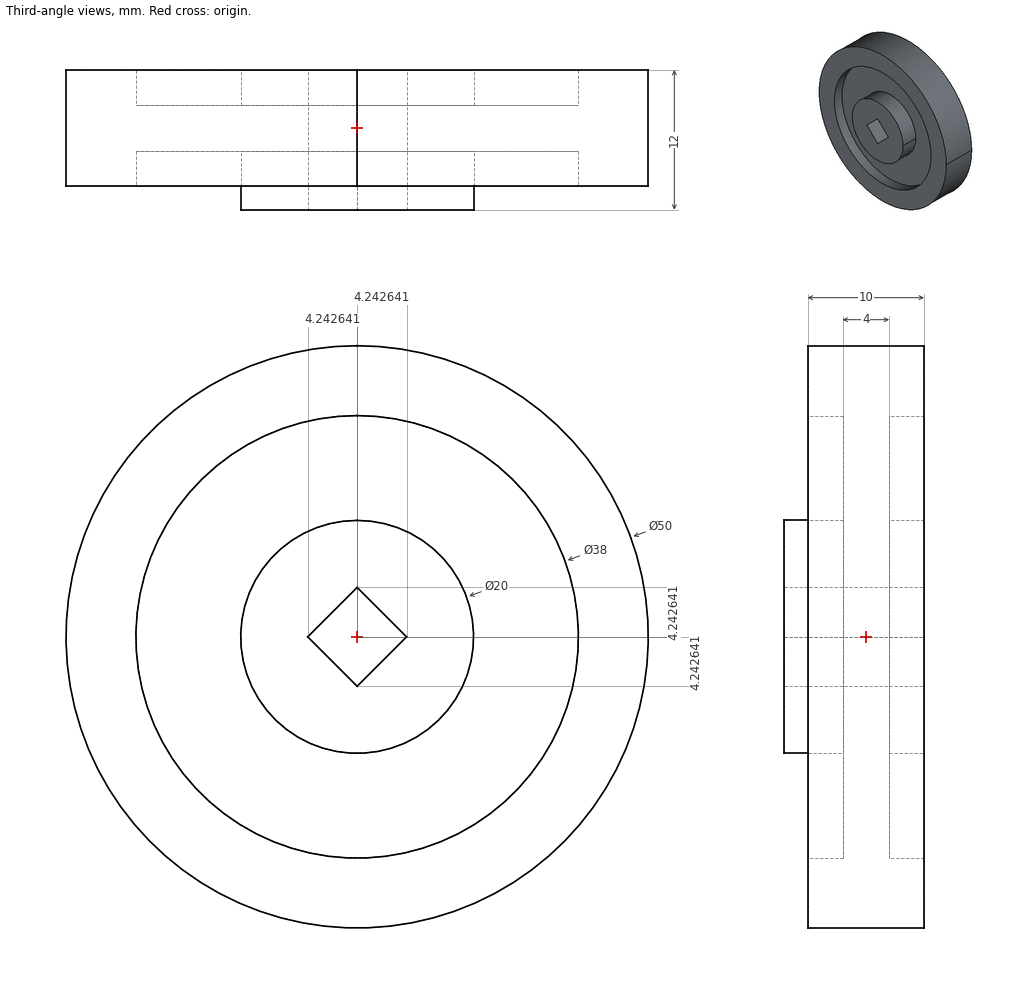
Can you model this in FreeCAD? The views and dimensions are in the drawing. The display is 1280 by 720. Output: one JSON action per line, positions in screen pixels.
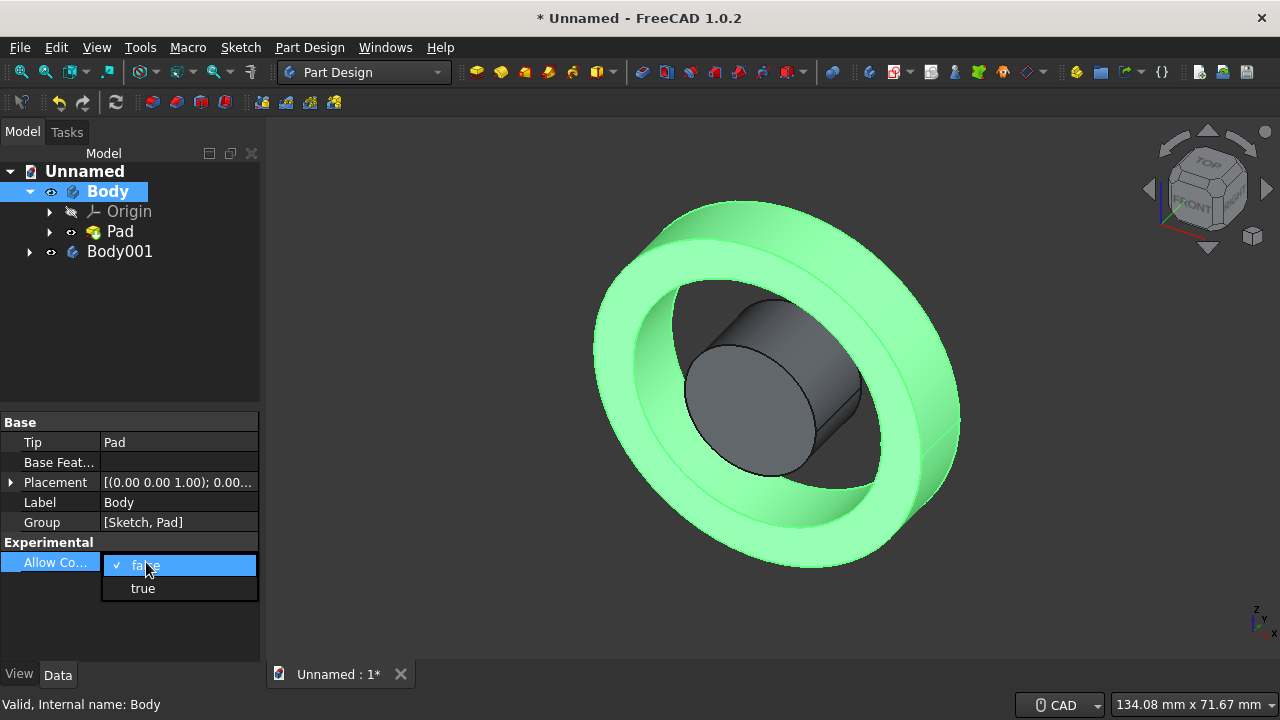
{"action": "left_click", "coordinate": [179, 588]}
{"action": "key", "text": "Return"}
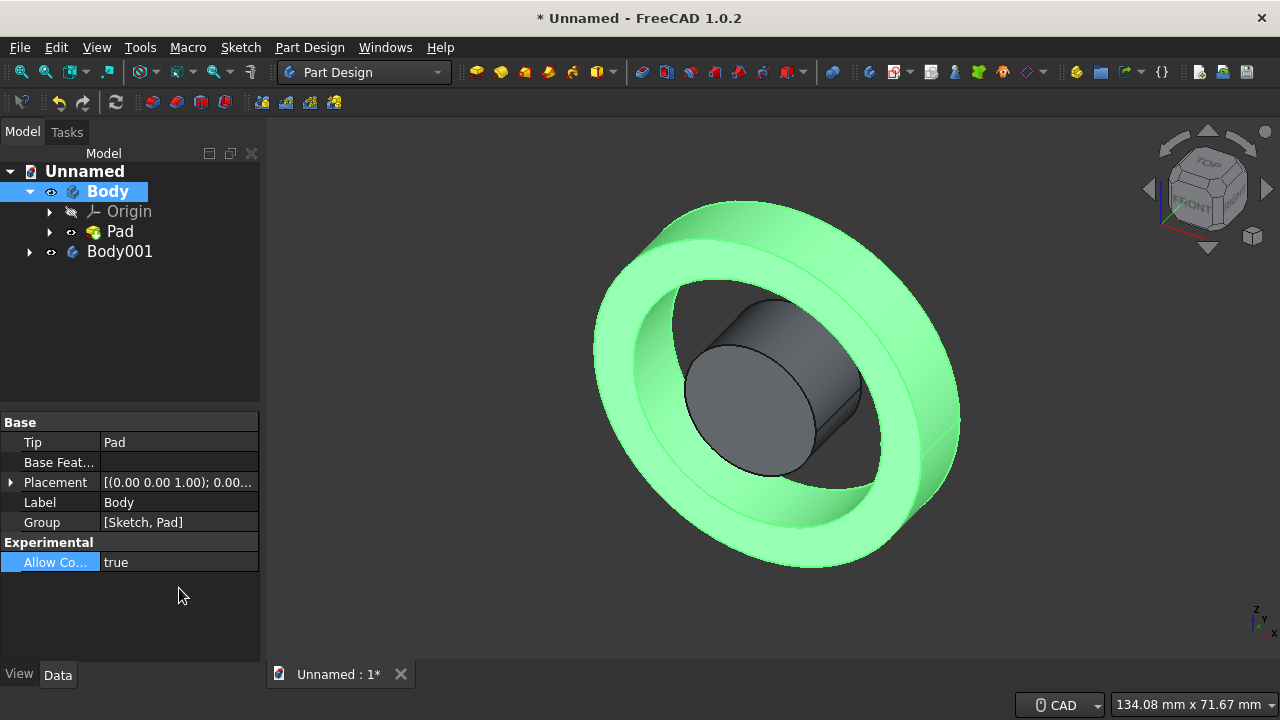
{"action": "left_click", "coordinate": [96, 252]}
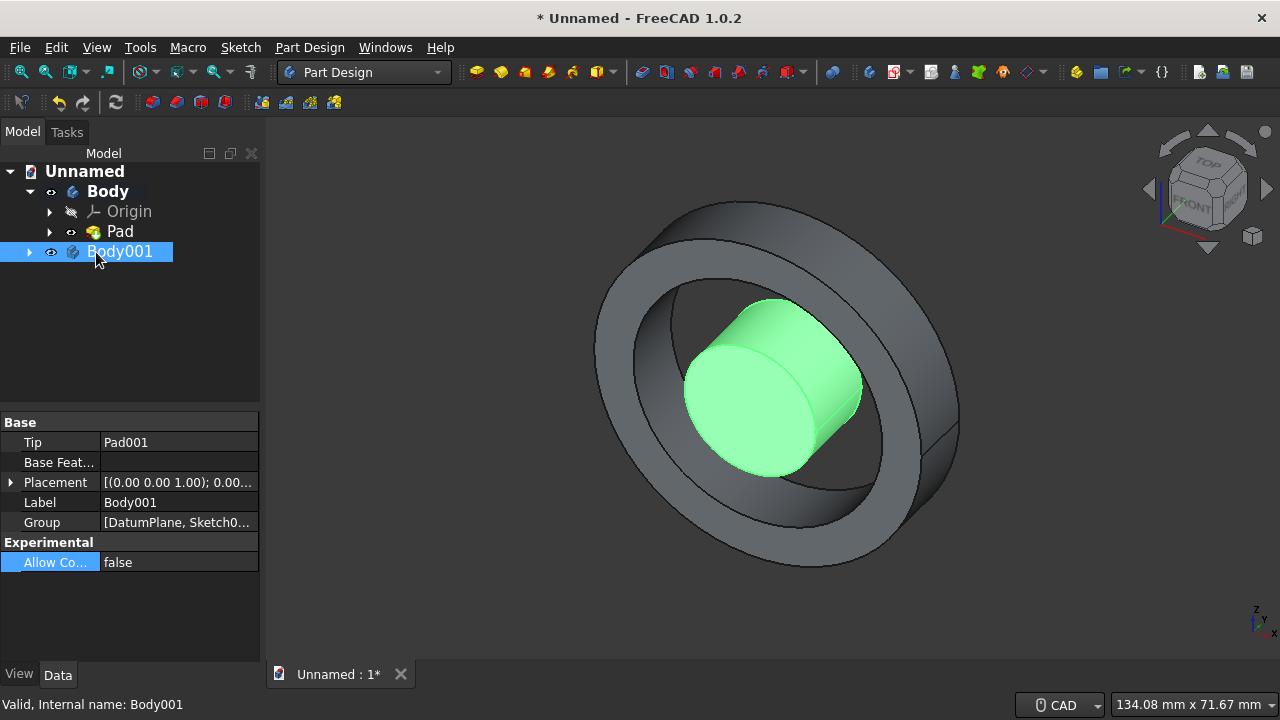
{"action": "left_click", "coordinate": [834, 72]}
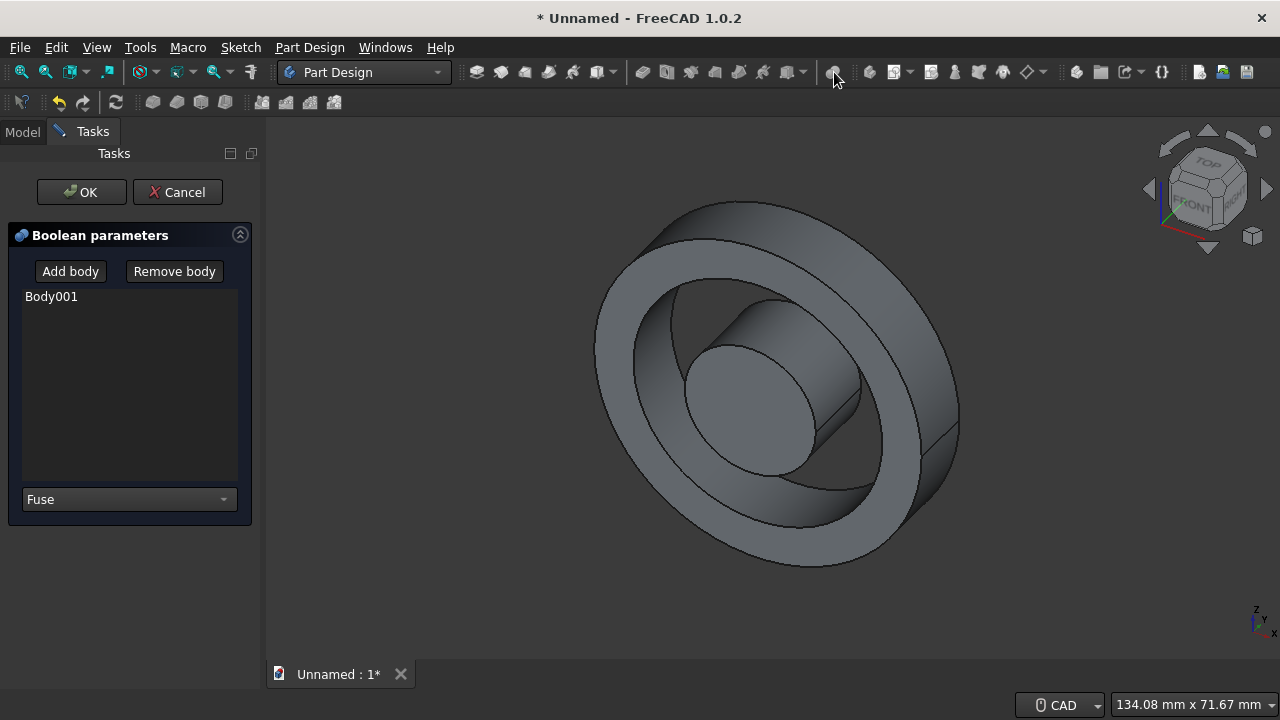
{"action": "left_click", "coordinate": [82, 192]}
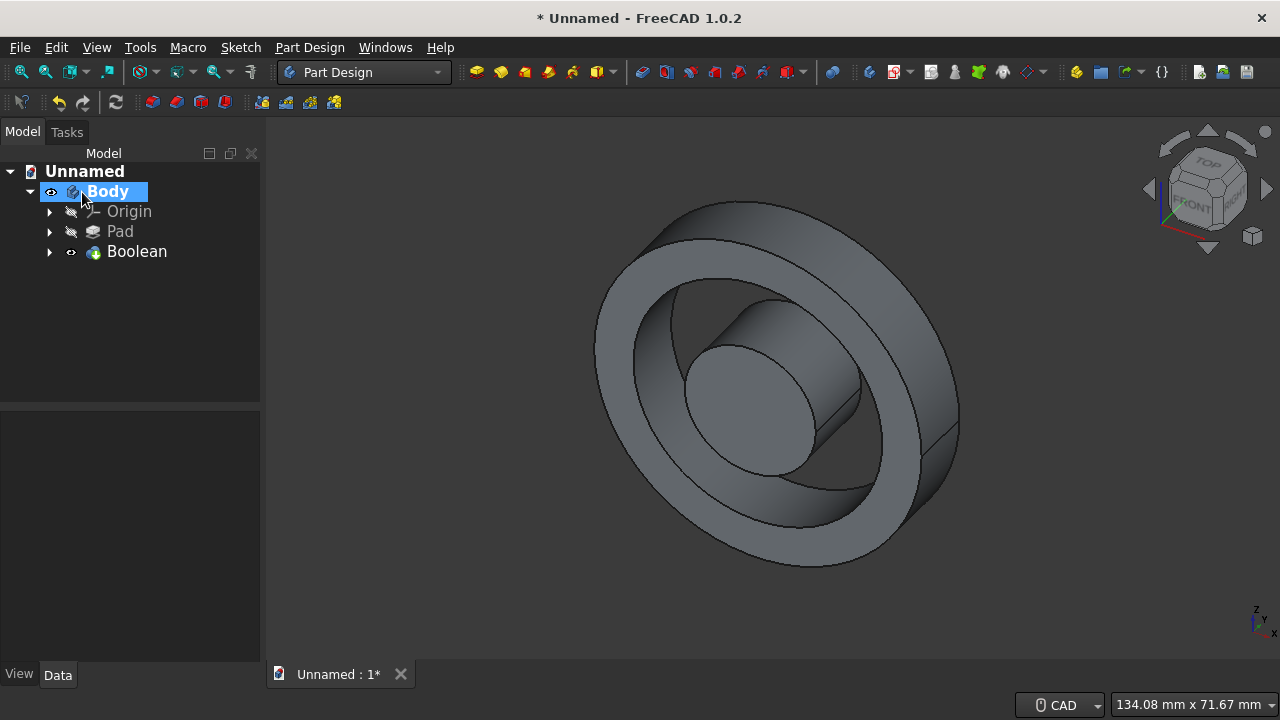
{"action": "left_click", "coordinate": [894, 72]}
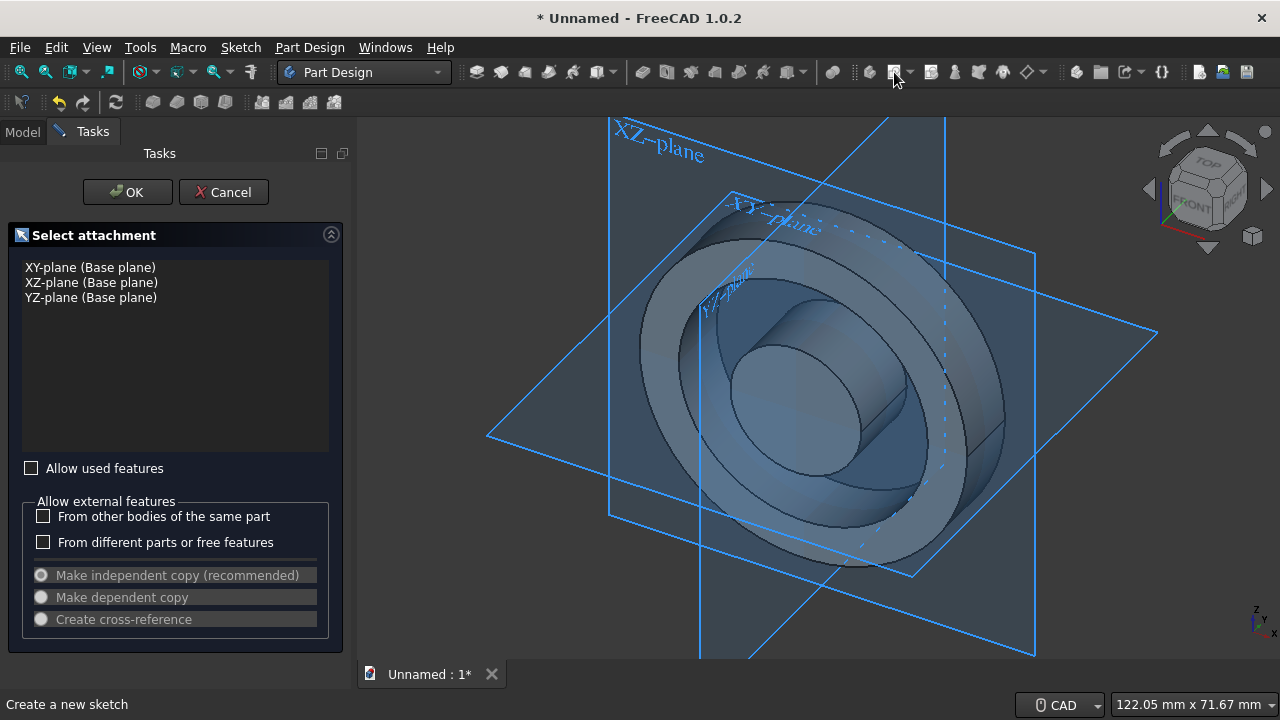
{"action": "left_click", "coordinate": [82, 282]}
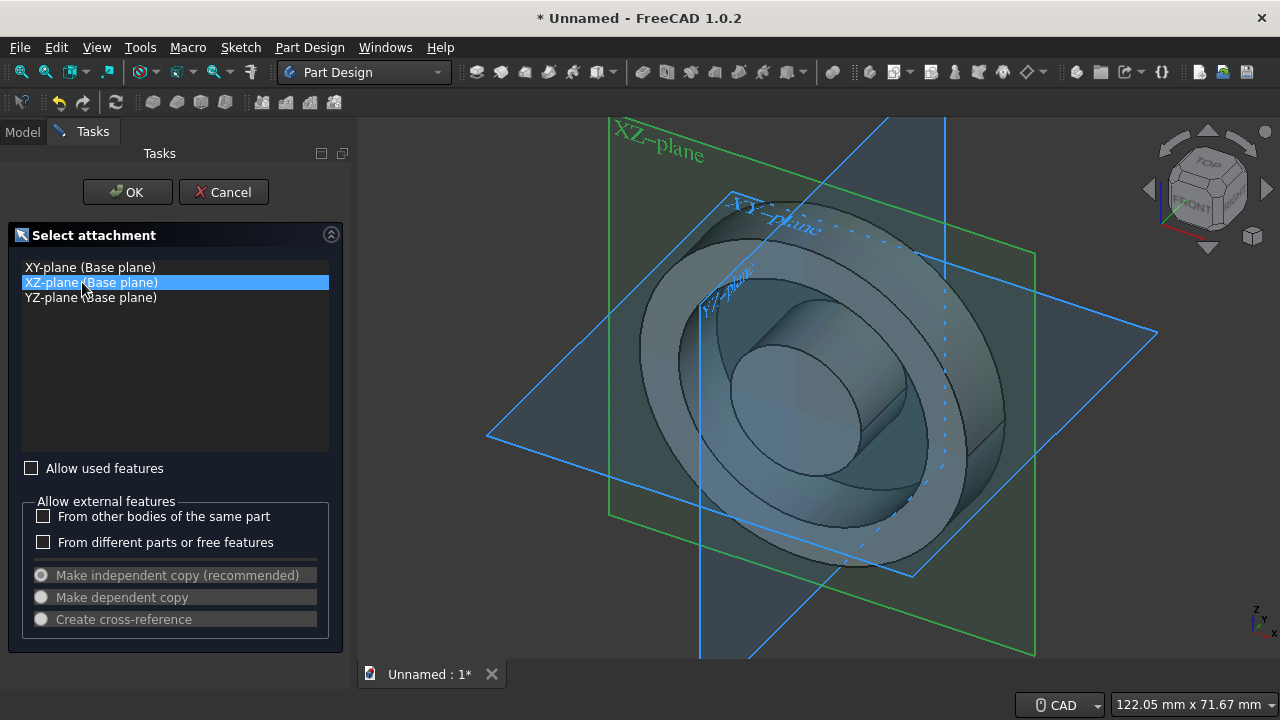
{"action": "left_click", "coordinate": [128, 192]}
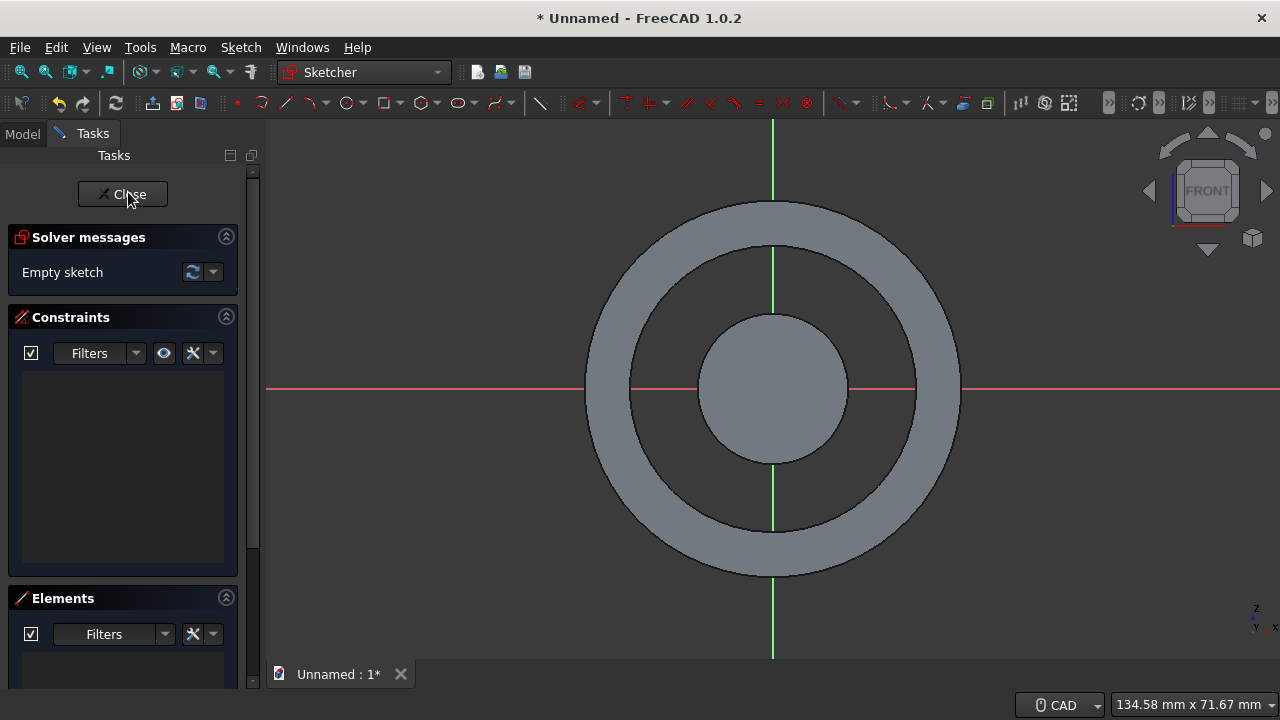
{"action": "left_click", "coordinate": [202, 104]}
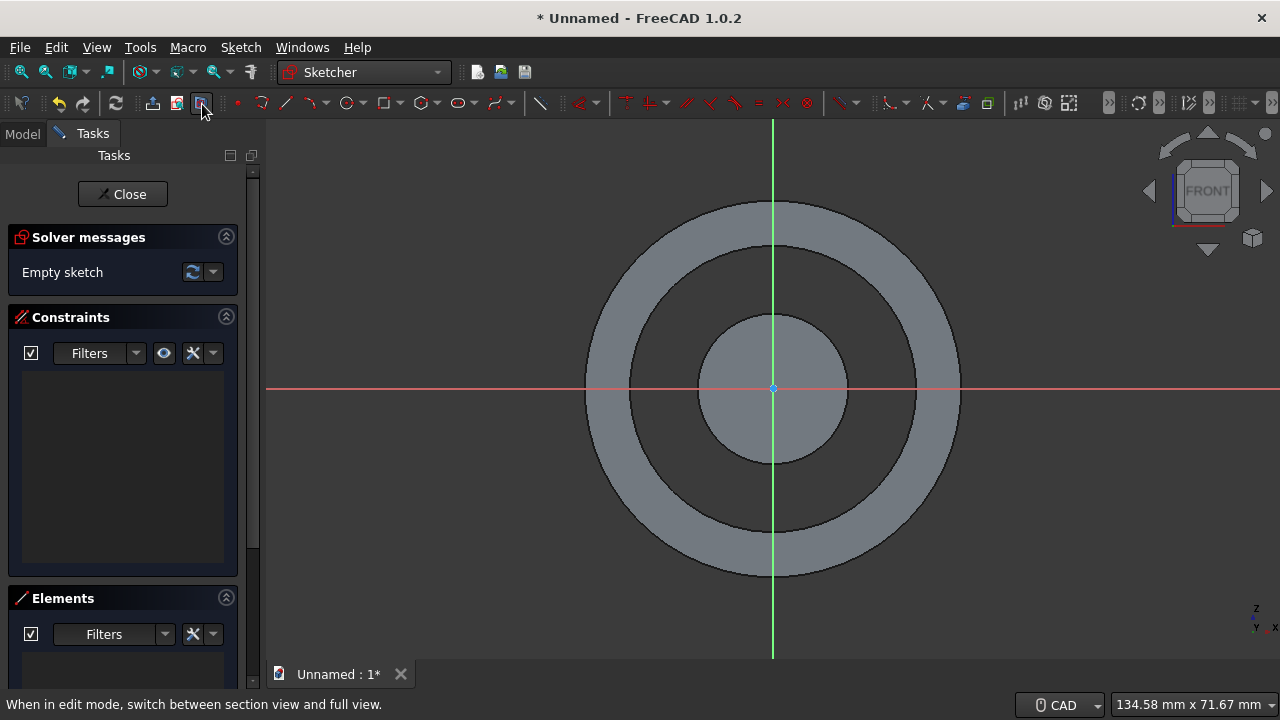
{"action": "left_click", "coordinate": [348, 104]}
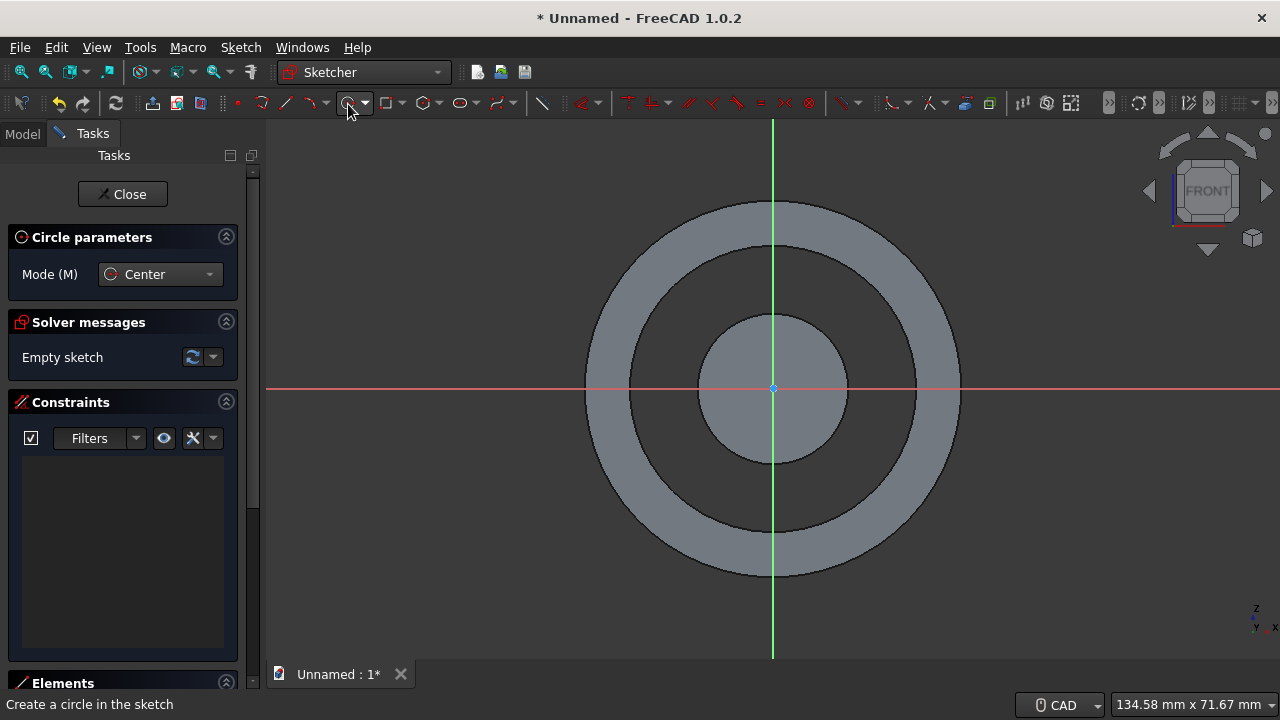
{"action": "left_click", "coordinate": [773, 389]}
{"action": "left_click", "coordinate": [874, 288]}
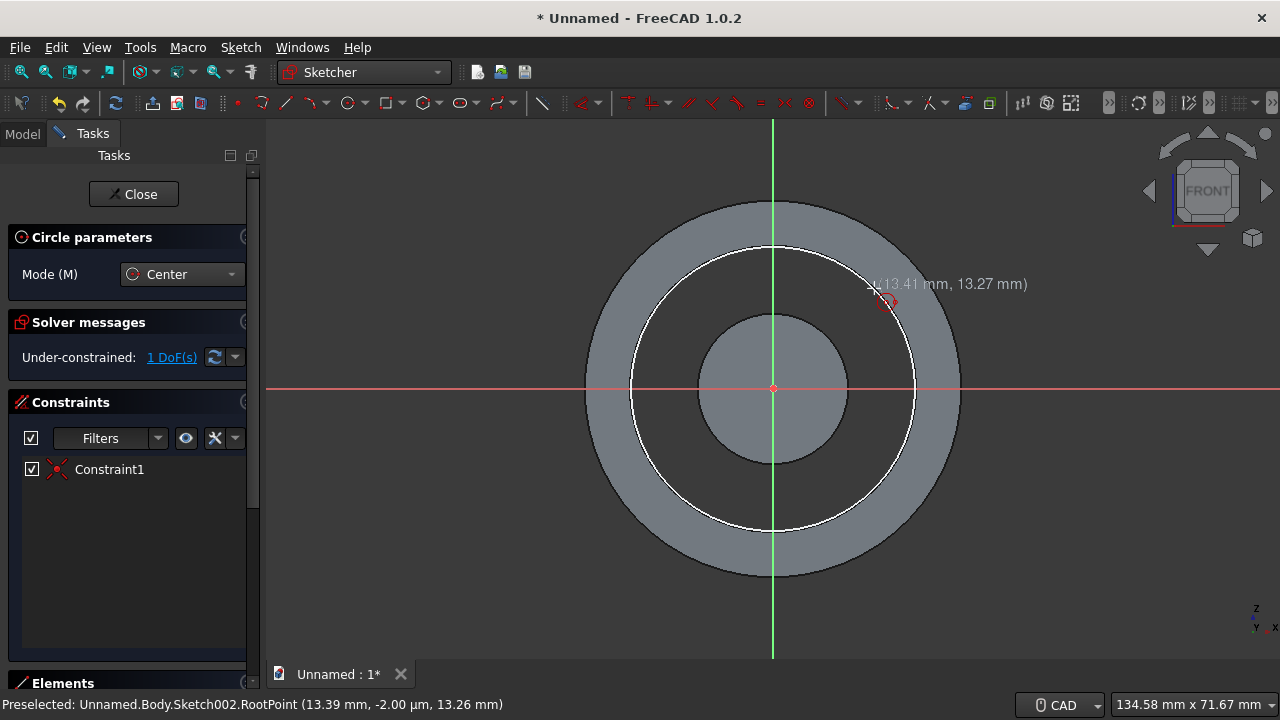
{"action": "left_click", "coordinate": [773, 389]}
{"action": "left_click", "coordinate": [826, 336]}
{"action": "key", "text": "Escape"}